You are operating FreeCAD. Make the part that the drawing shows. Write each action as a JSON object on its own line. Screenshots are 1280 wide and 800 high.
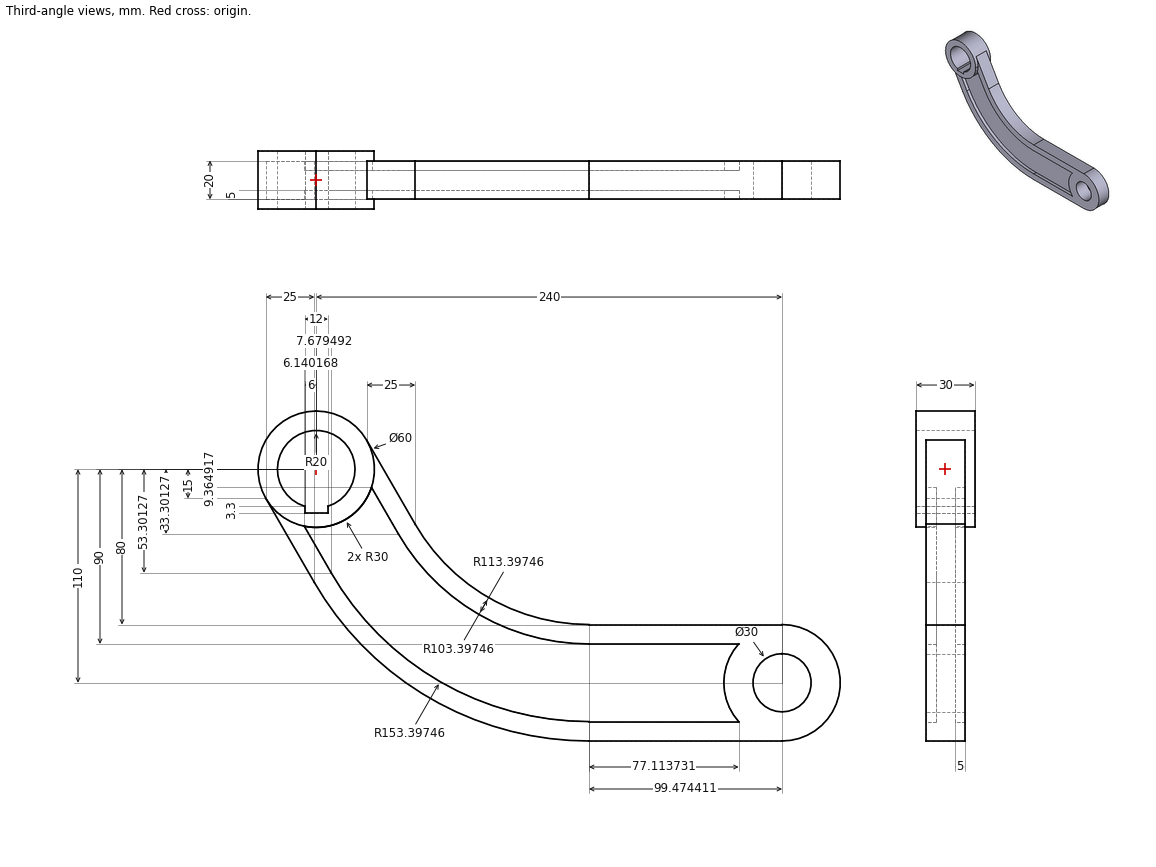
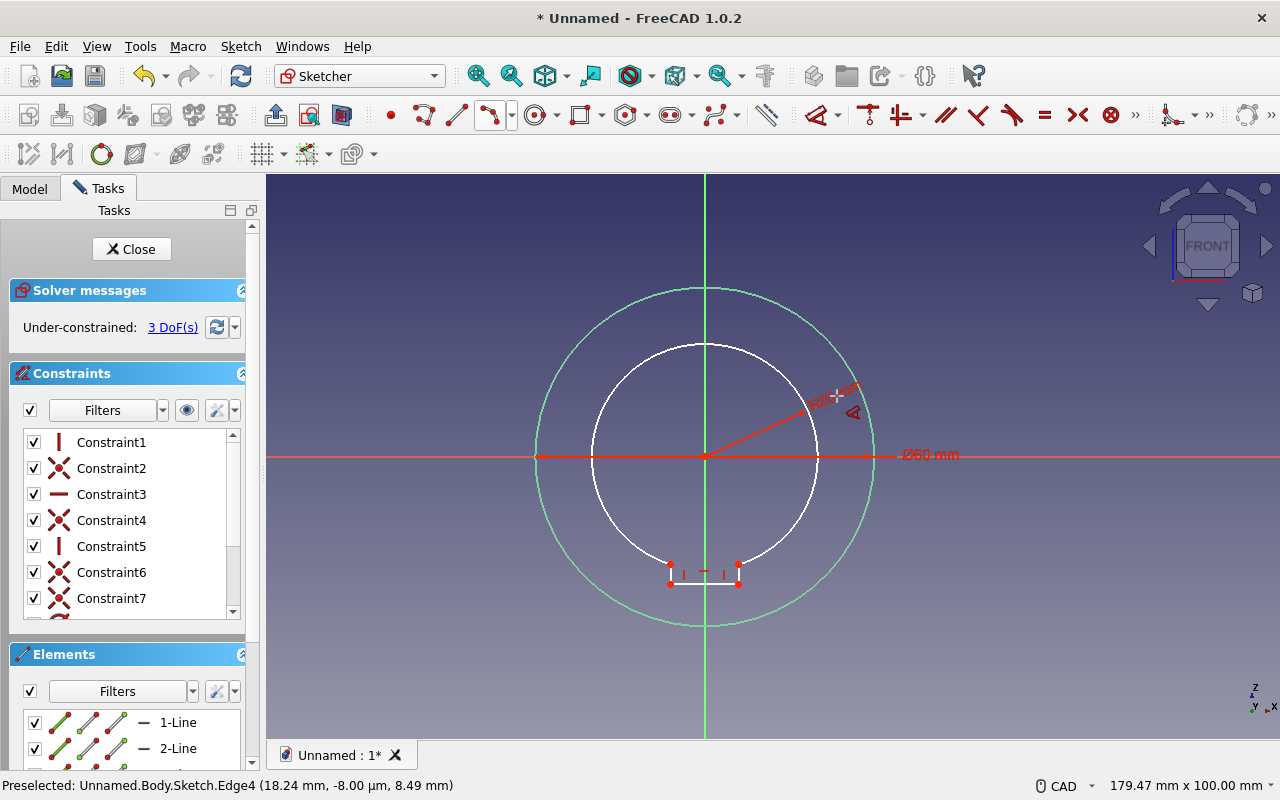
{"action": "left_click", "coordinate": [691, 584]}
{"action": "left_click", "coordinate": [689, 550]}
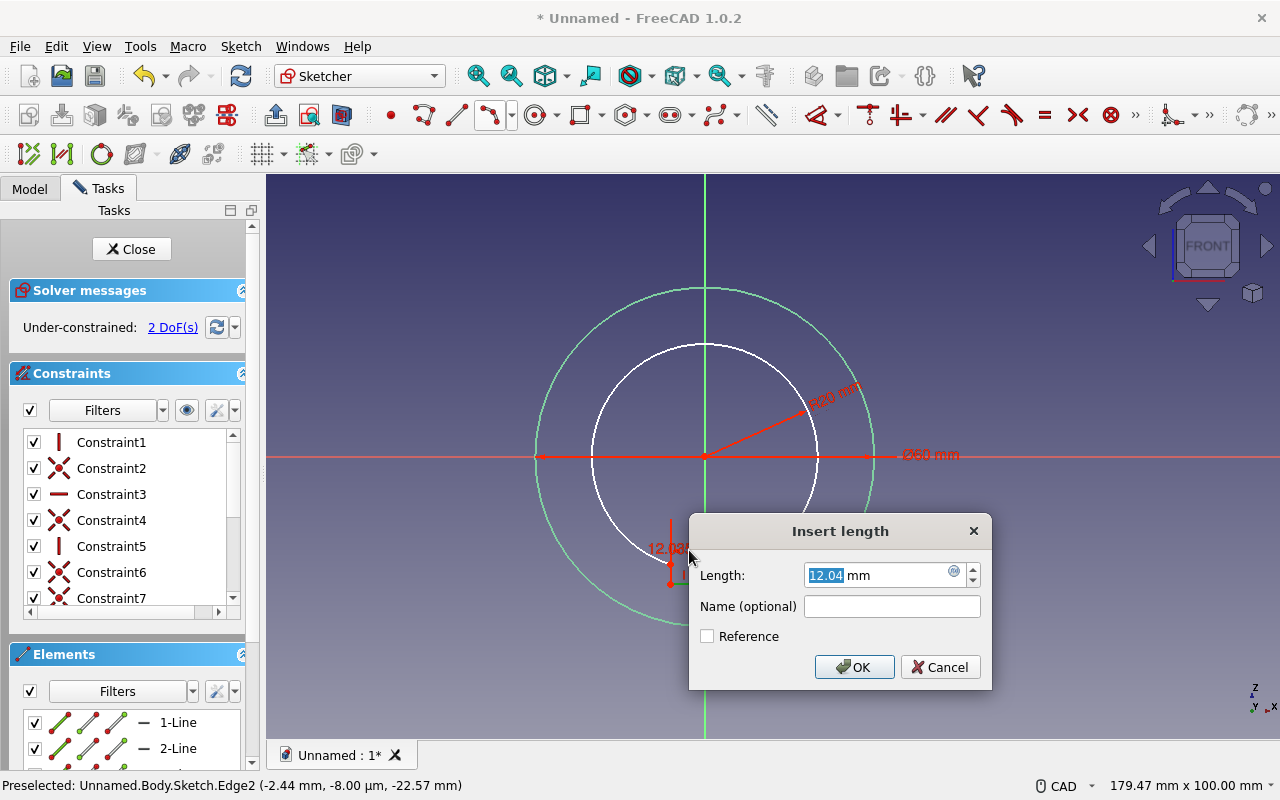
{"action": "type", "text": "12"}
{"action": "key", "text": "Return"}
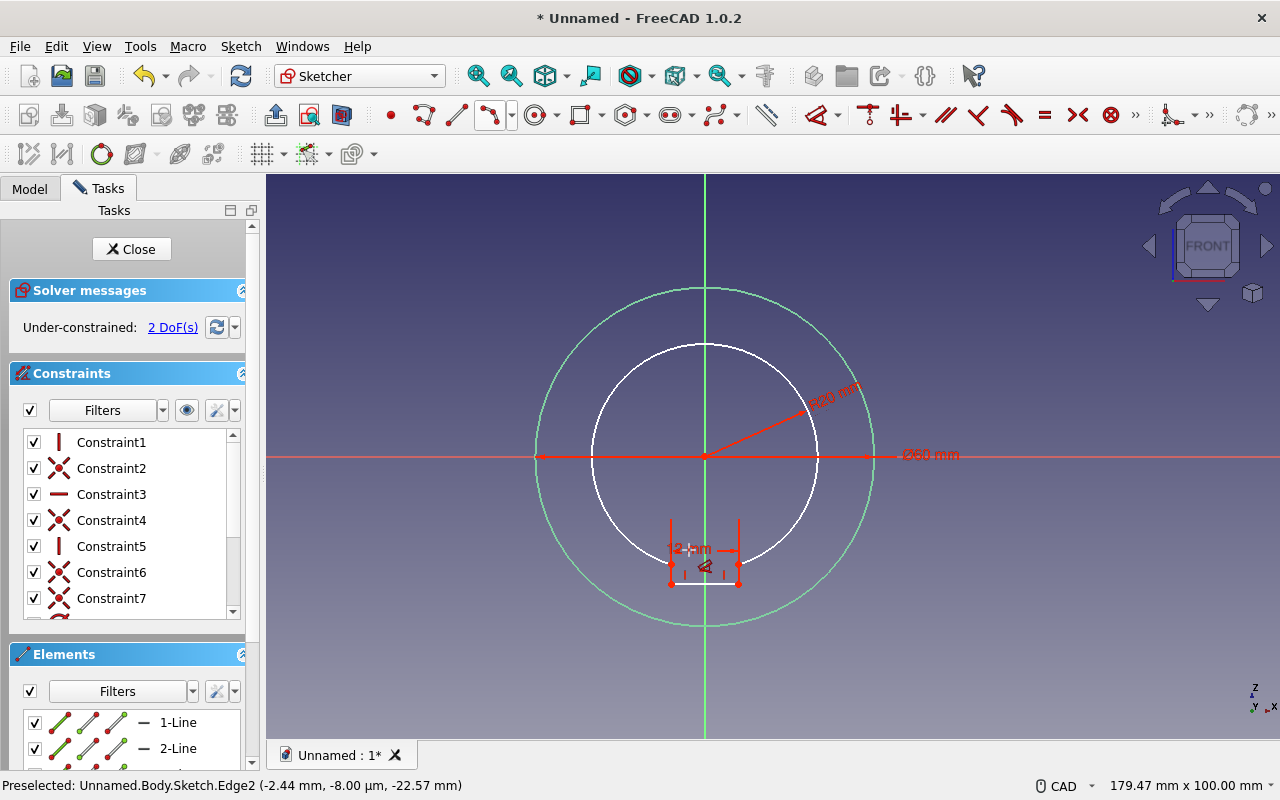
{"action": "left_click", "coordinate": [671, 565]}
{"action": "left_click", "coordinate": [688, 599]}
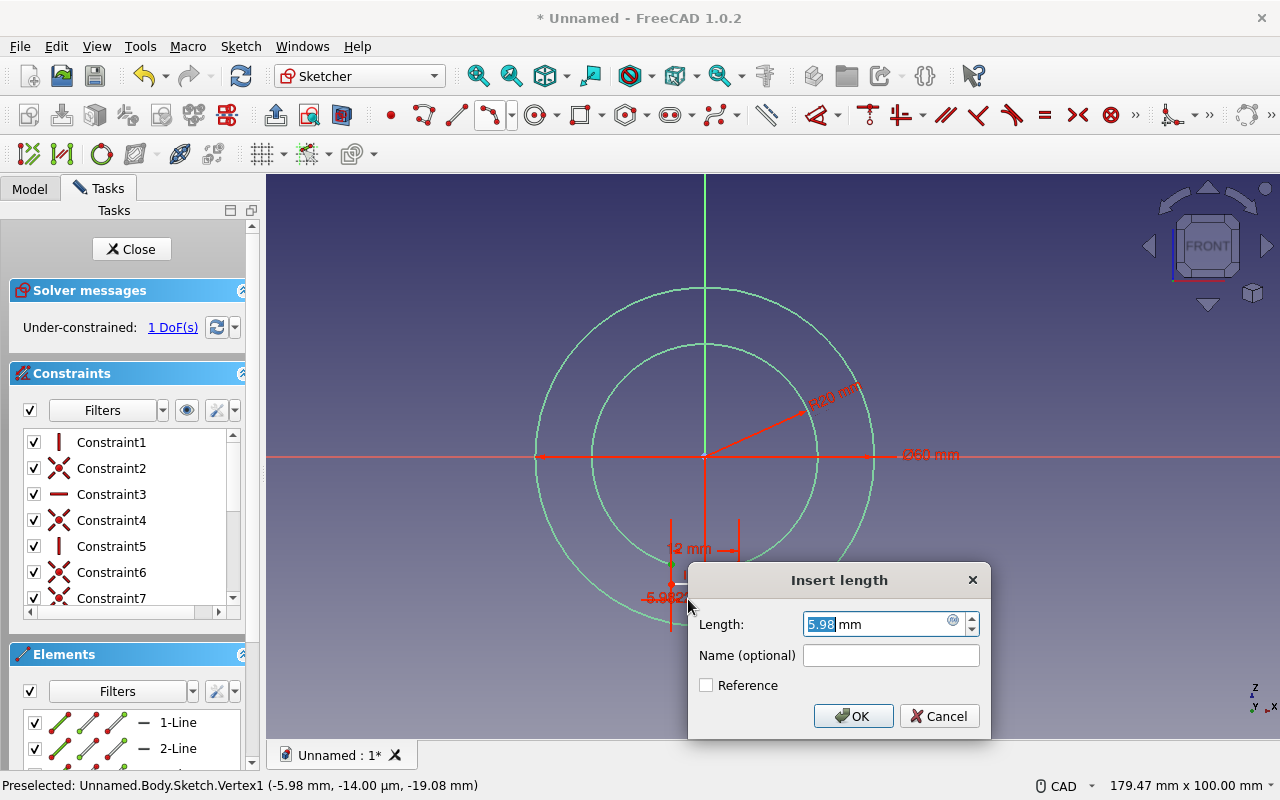
{"action": "type", "text": "6"}
{"action": "key", "text": "Return"}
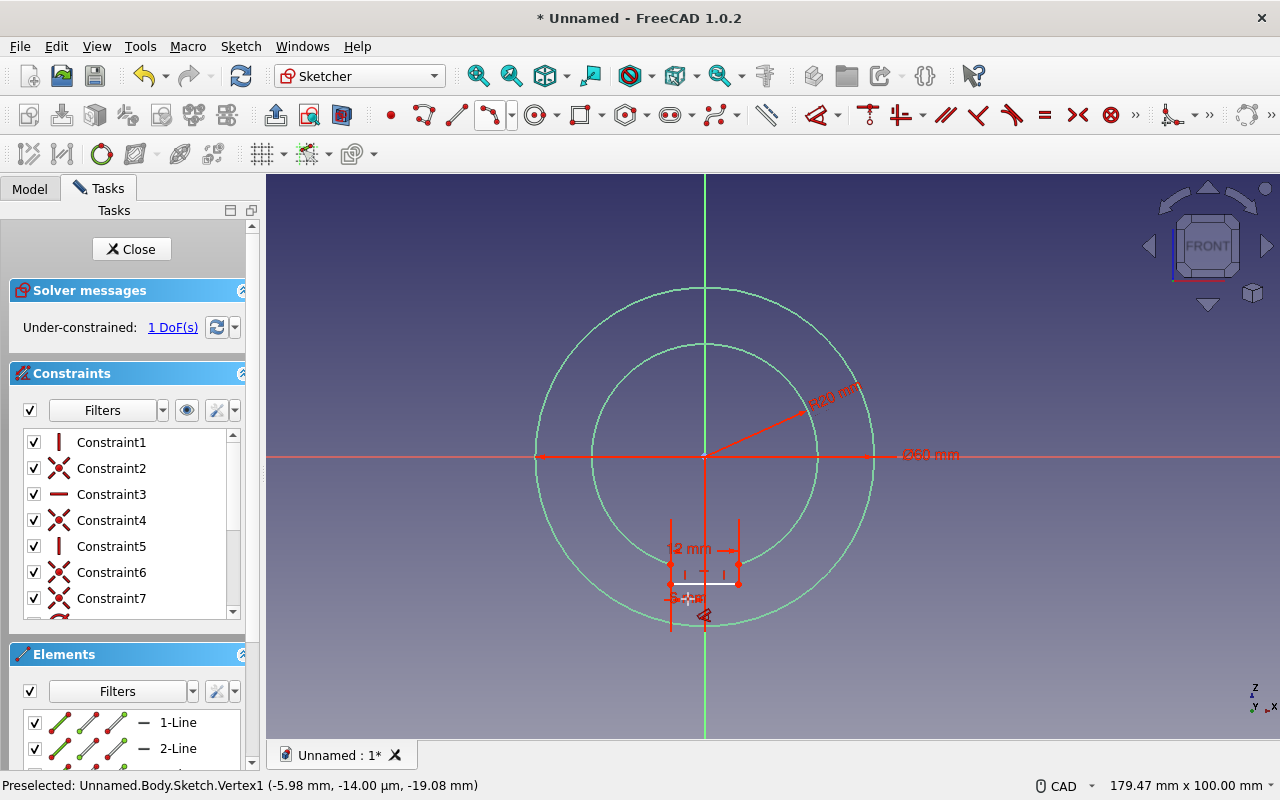
{"action": "scroll", "coordinate": [671, 575], "scroll_direction": "up", "scroll_amount": 4}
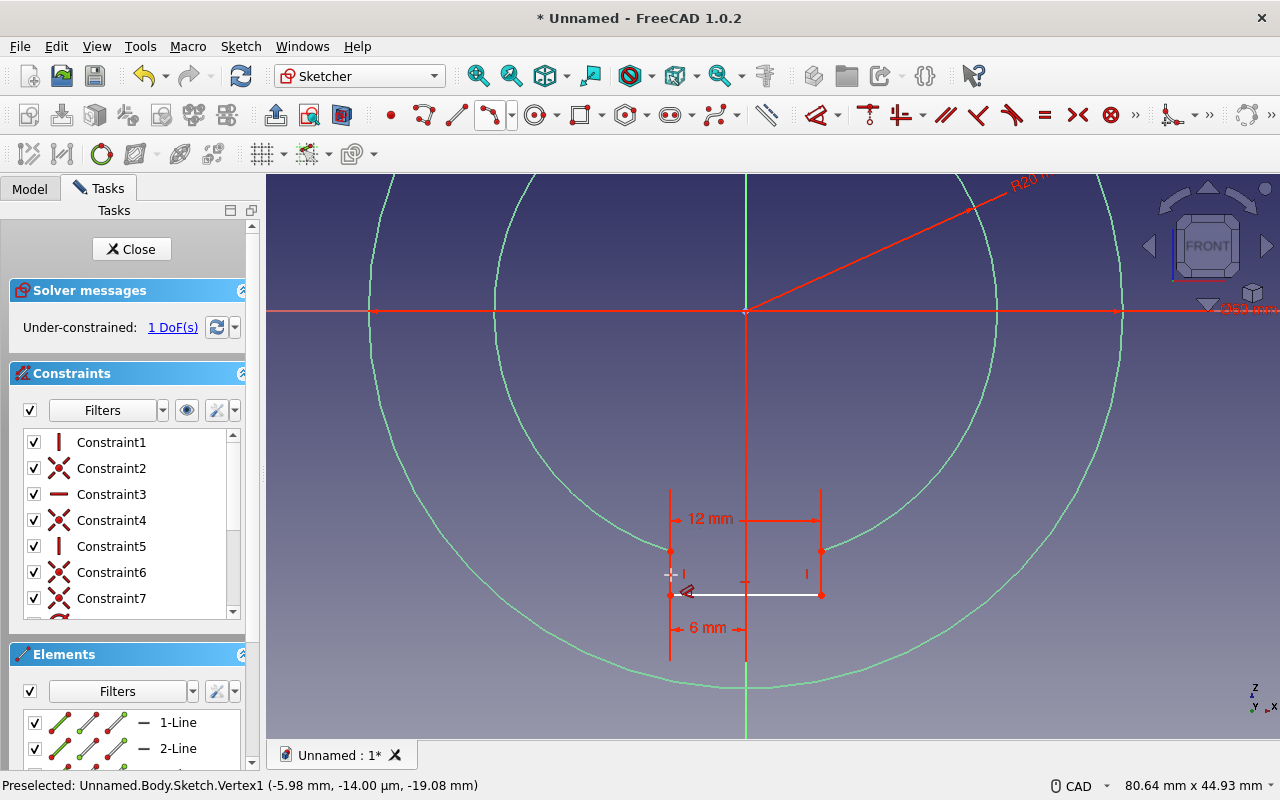
{"action": "left_click", "coordinate": [670, 573]}
{"action": "left_click", "coordinate": [636, 573]}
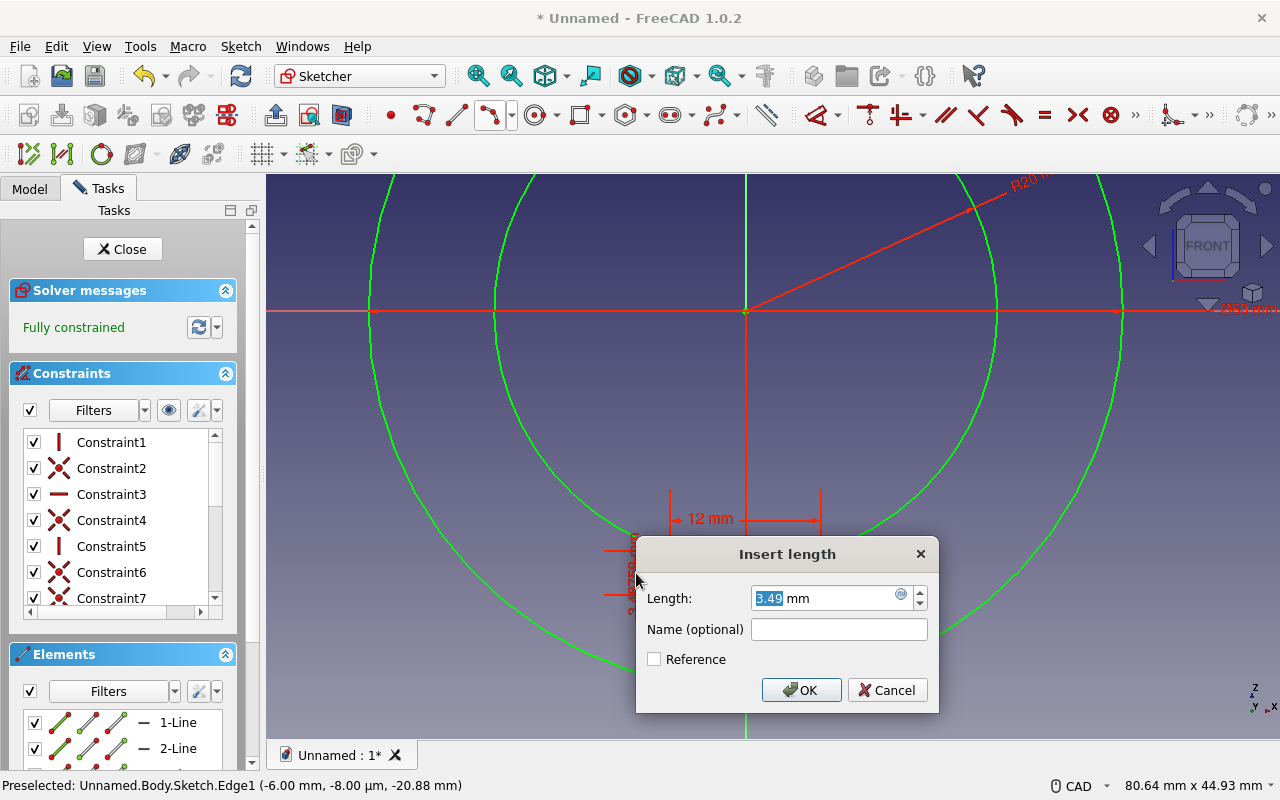
{"action": "type", "text": "3.3"}
{"action": "key", "text": "Return"}
{"action": "key", "text": "Escape"}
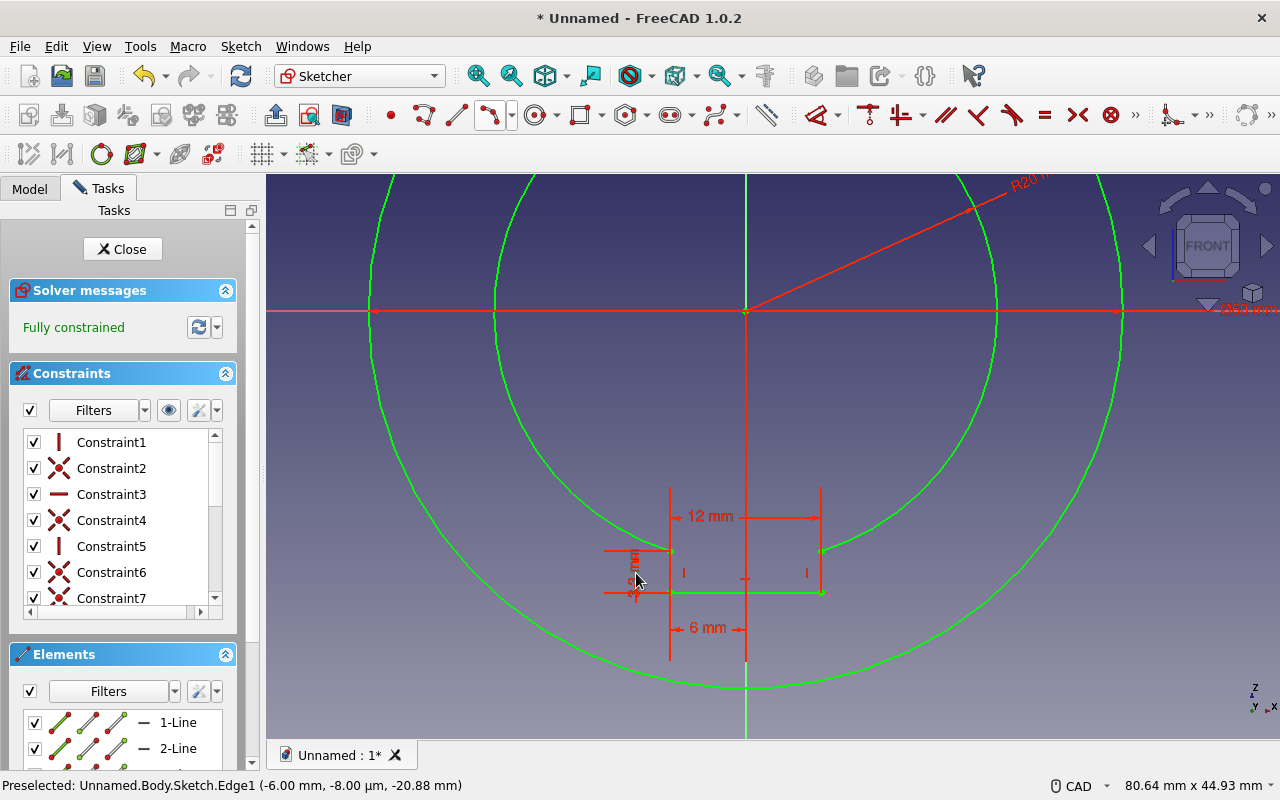
{"action": "left_click", "coordinate": [123, 249]}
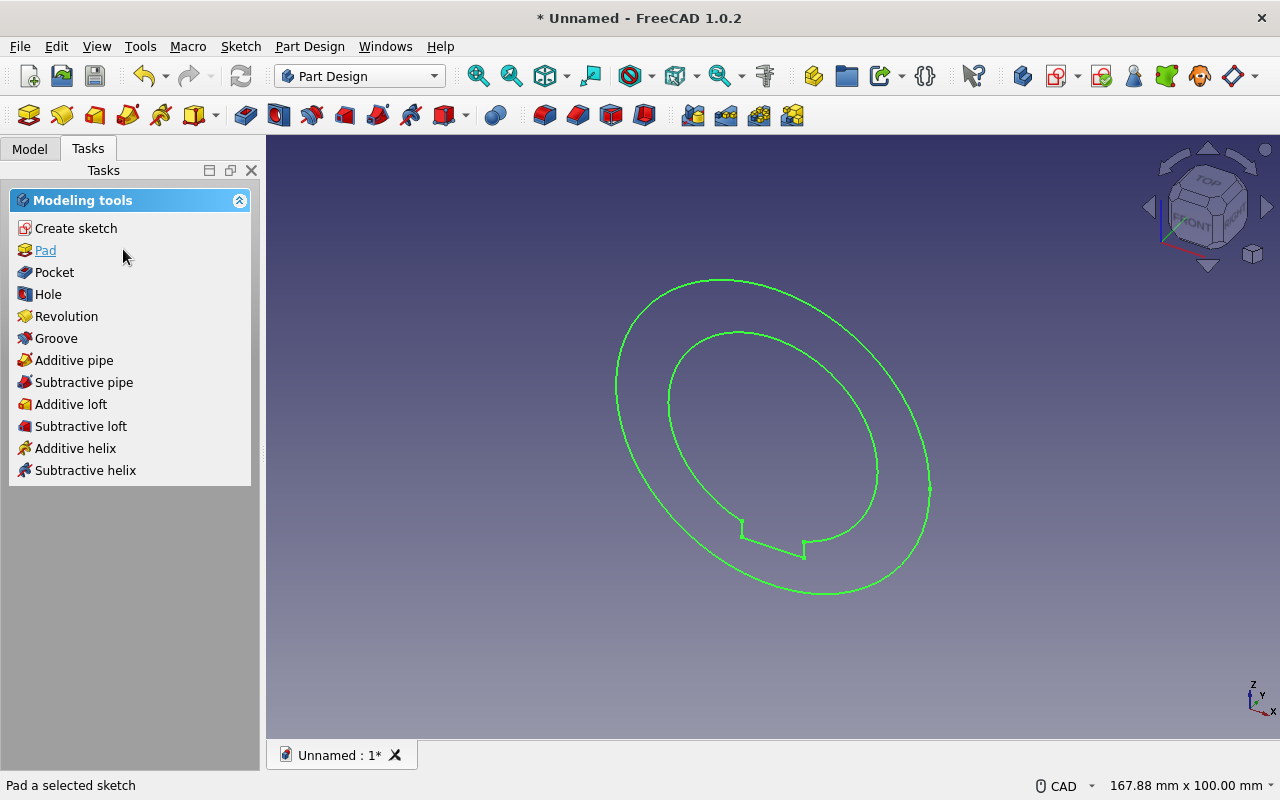
{"action": "left_click", "coordinate": [29, 116]}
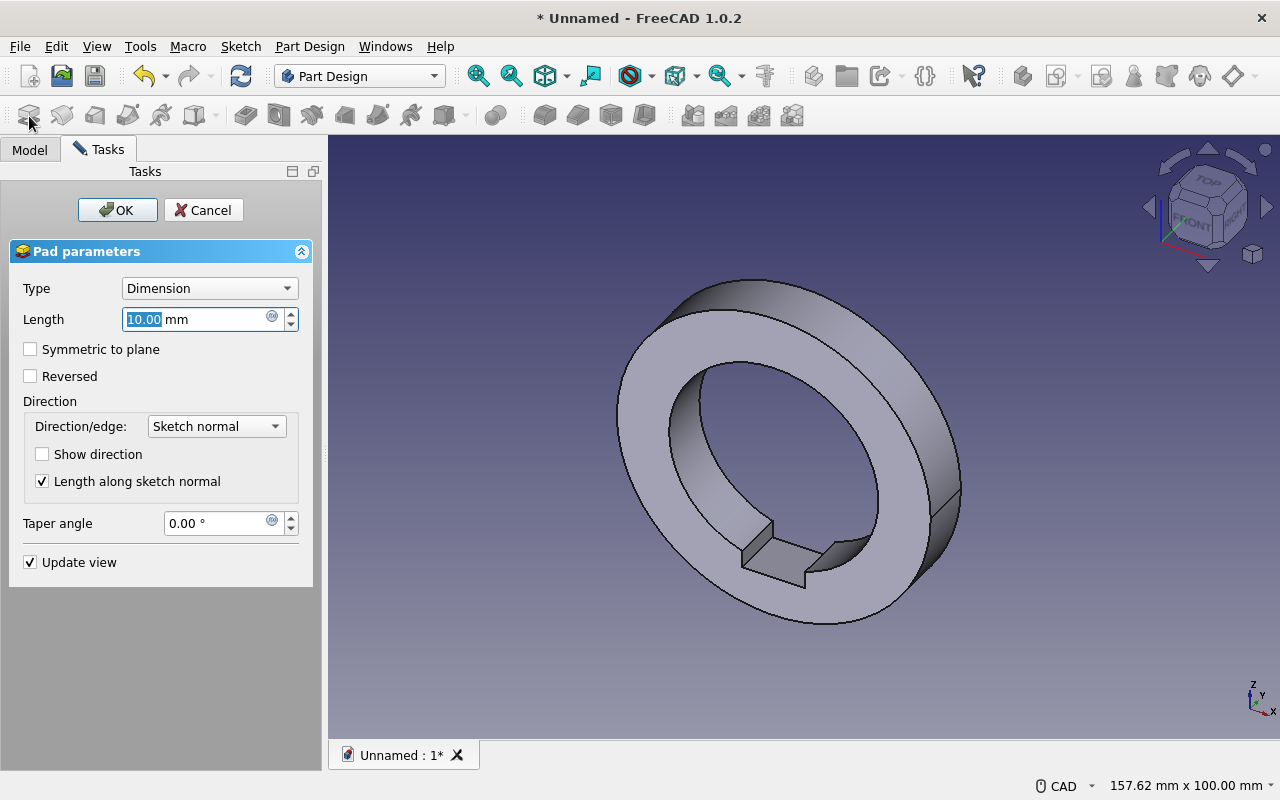
{"action": "type", "text": "30"}
{"action": "key", "text": "Tab"}